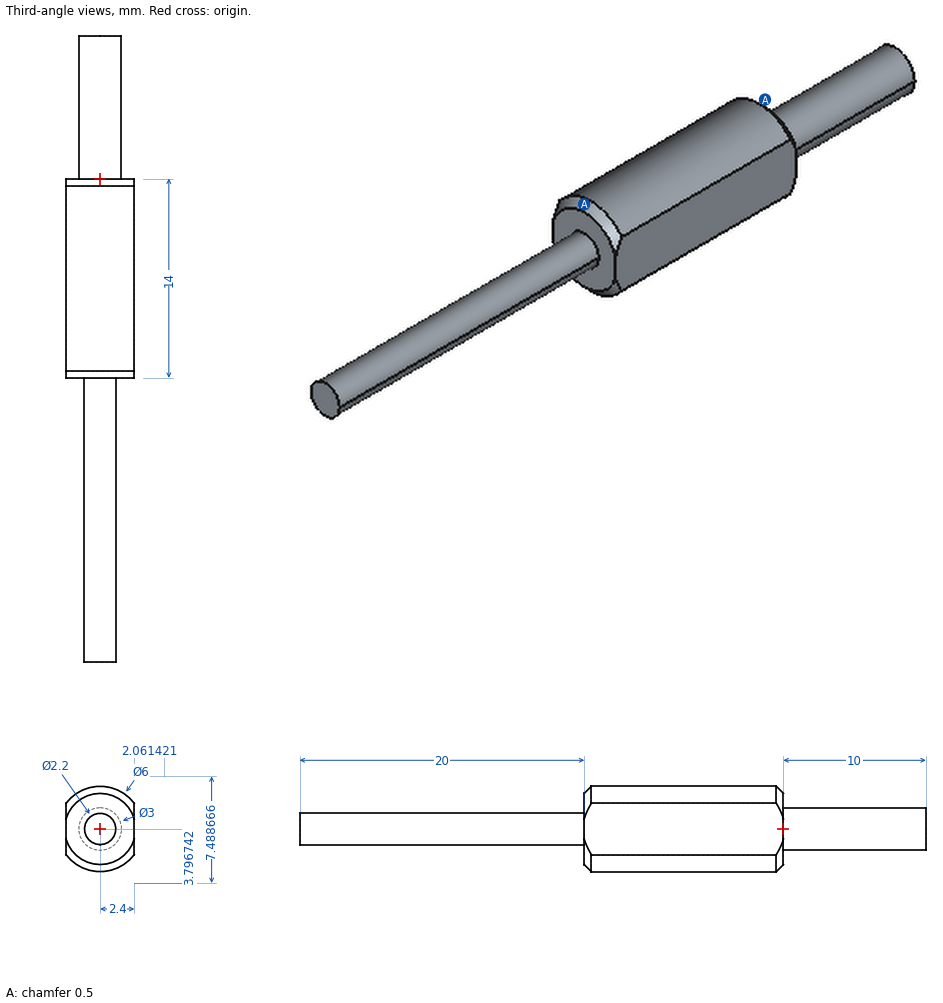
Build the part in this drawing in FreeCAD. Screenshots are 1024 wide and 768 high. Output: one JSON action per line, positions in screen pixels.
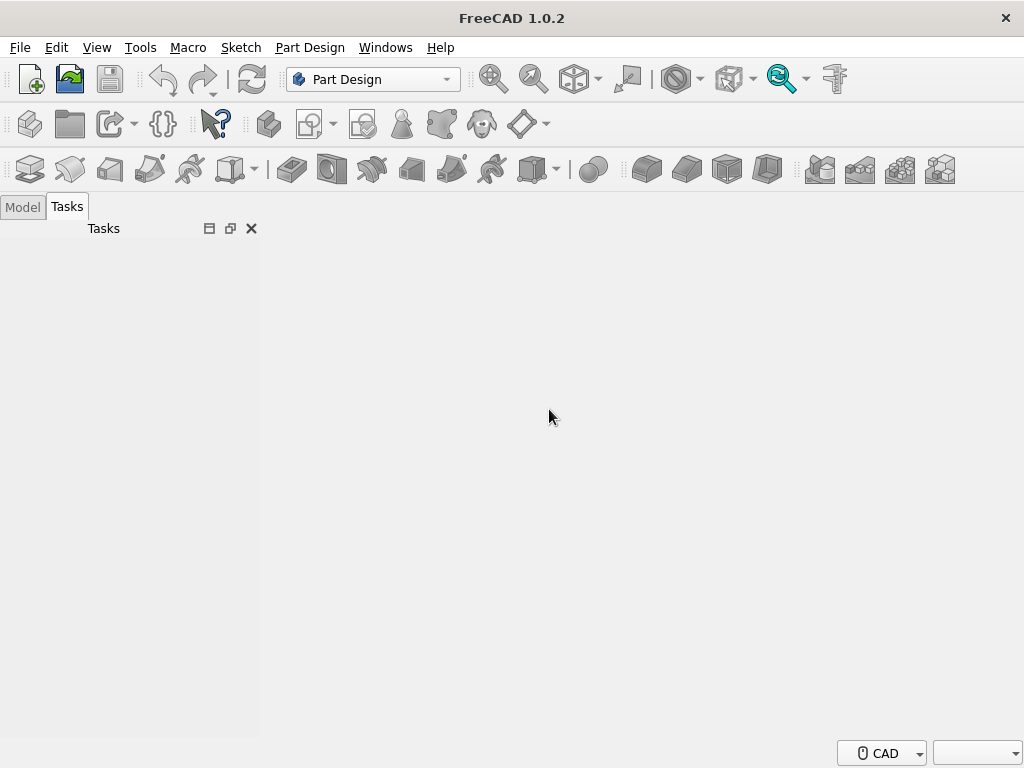
{"action": "key", "text": "ctrl+n"}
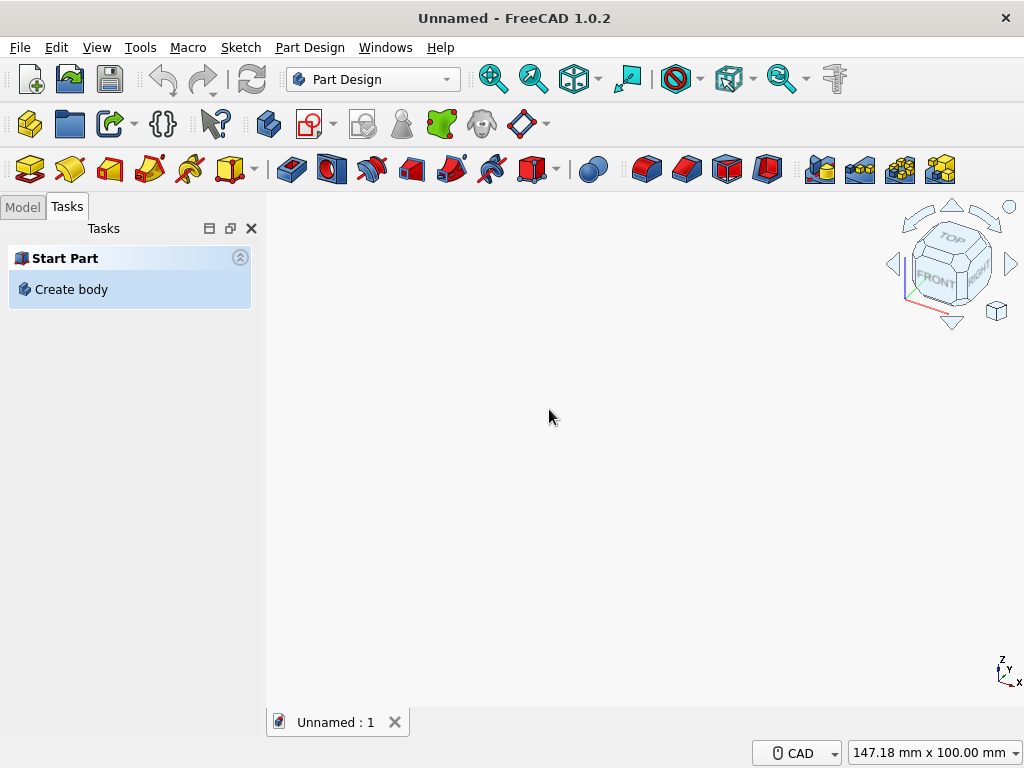
{"action": "left_click", "coordinate": [310, 124]}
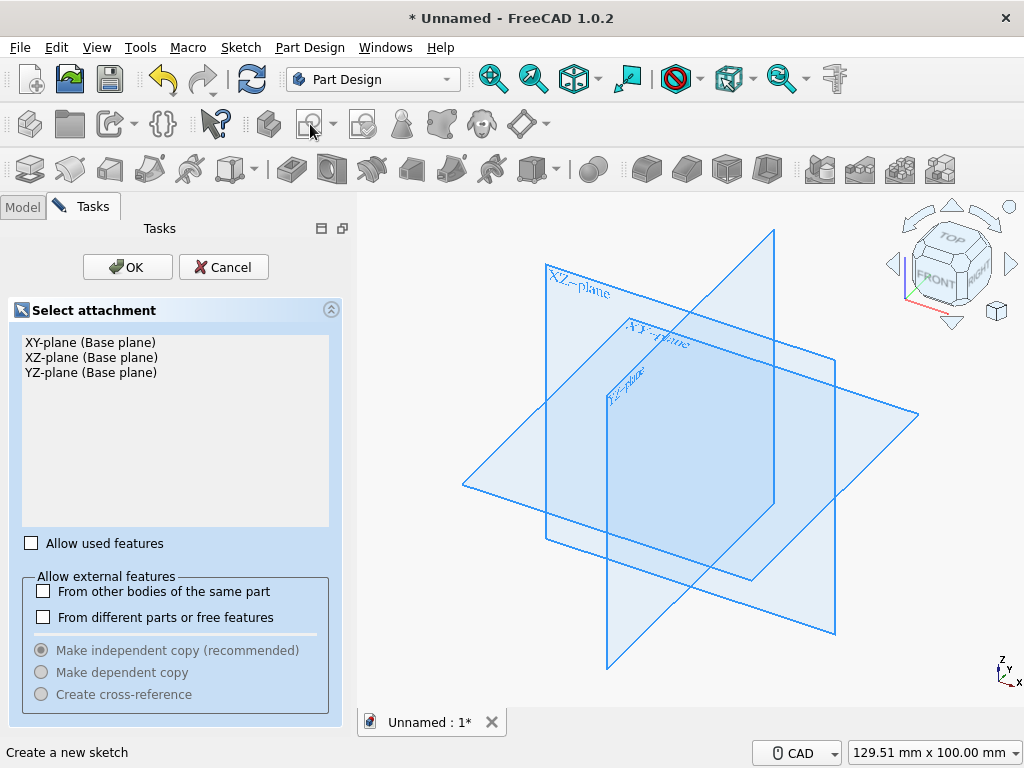
{"action": "left_click", "coordinate": [82, 358]}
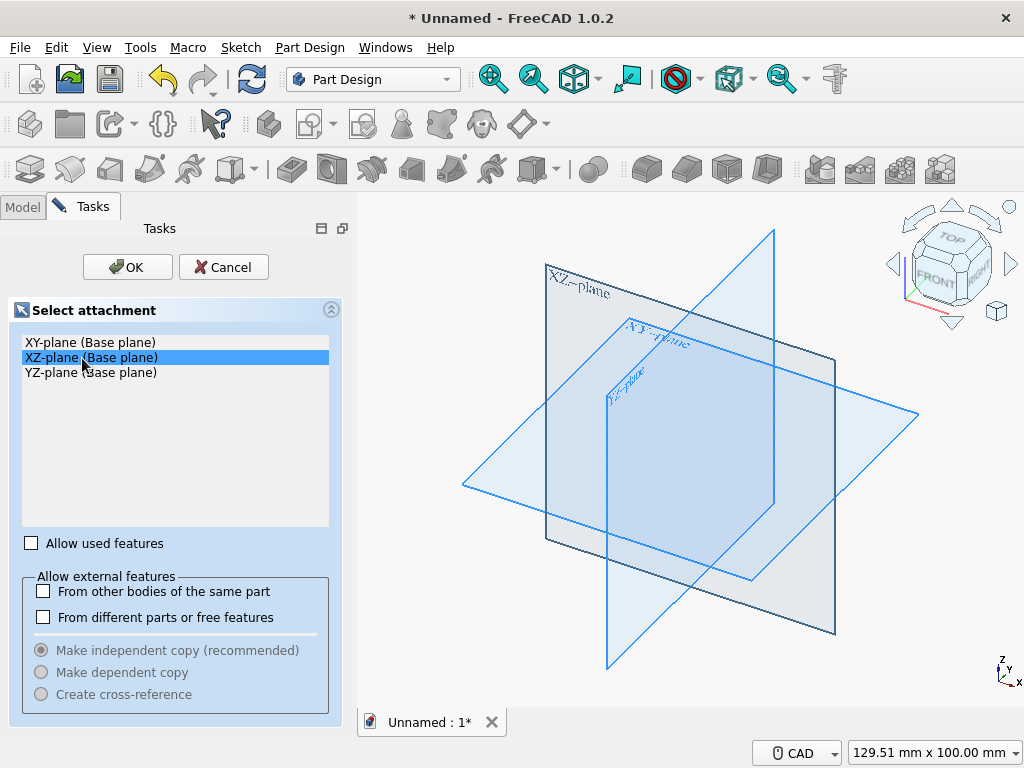
{"action": "left_click", "coordinate": [128, 267]}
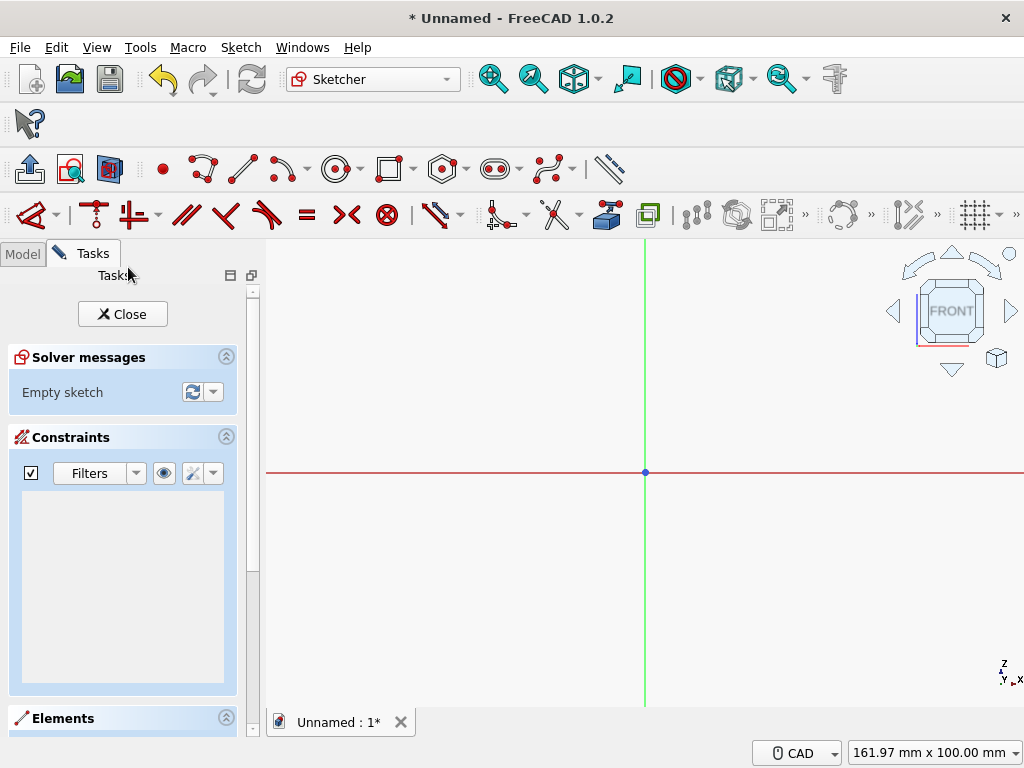
{"action": "scroll", "coordinate": [649, 473], "scroll_direction": "up", "scroll_amount": 15}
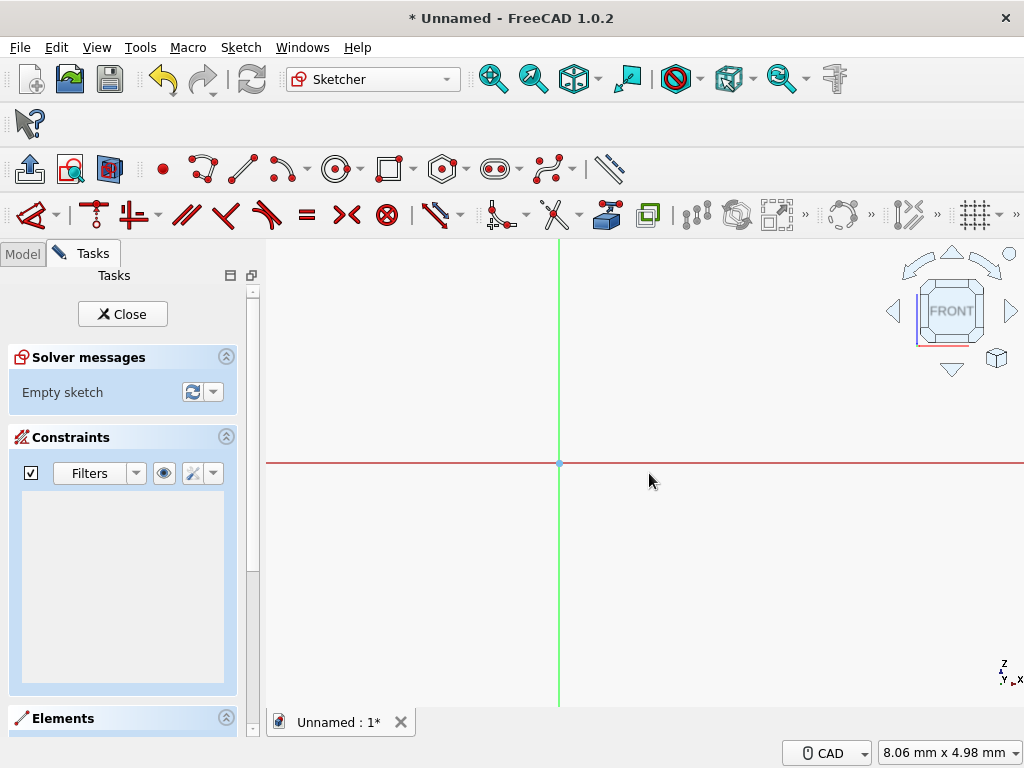
{"action": "left_click", "coordinate": [336, 170]}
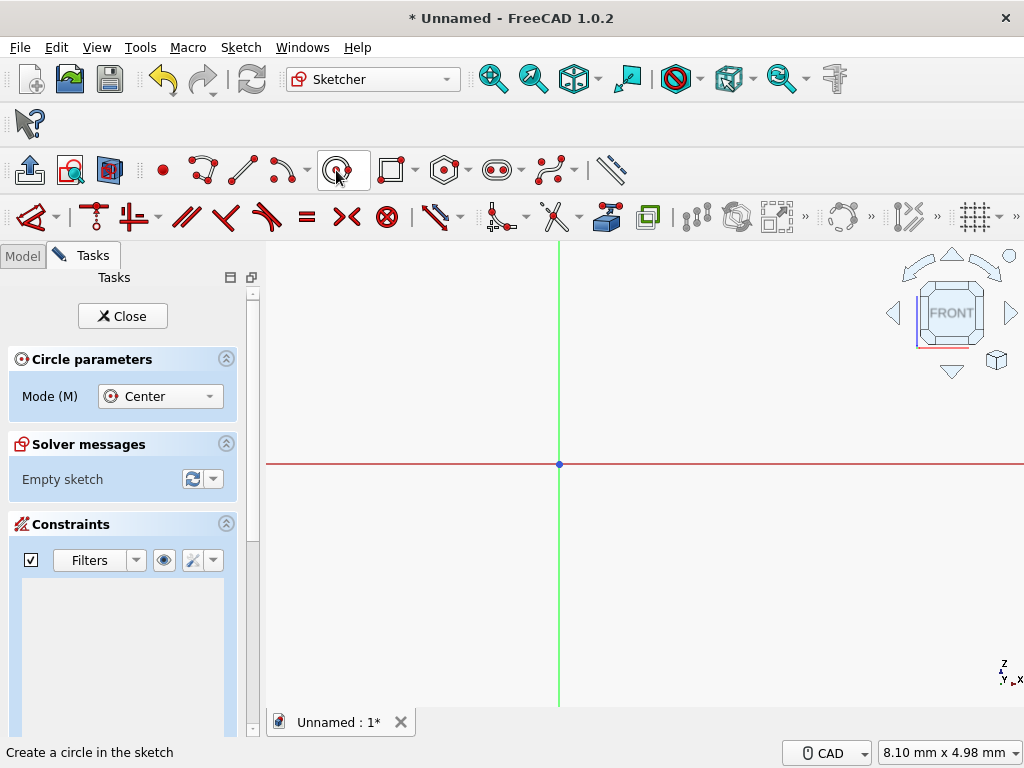
{"action": "left_click", "coordinate": [559, 464]}
{"action": "left_click", "coordinate": [659, 365]}
{"action": "key", "text": "Escape"}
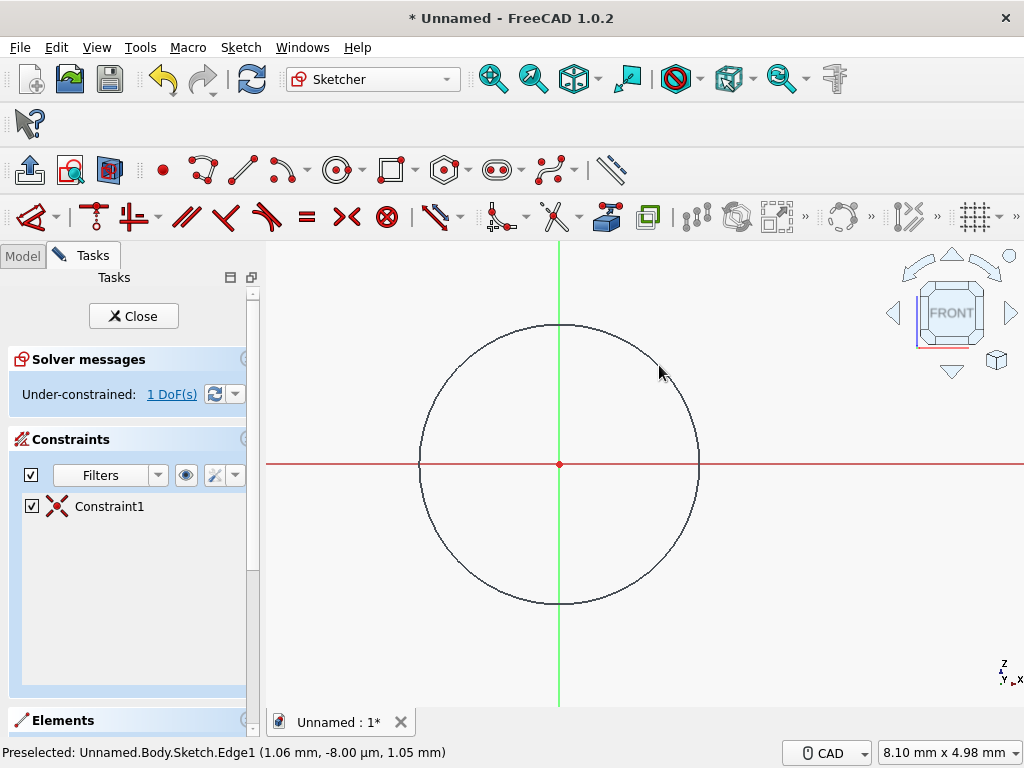
{"action": "left_click", "coordinate": [32, 218]}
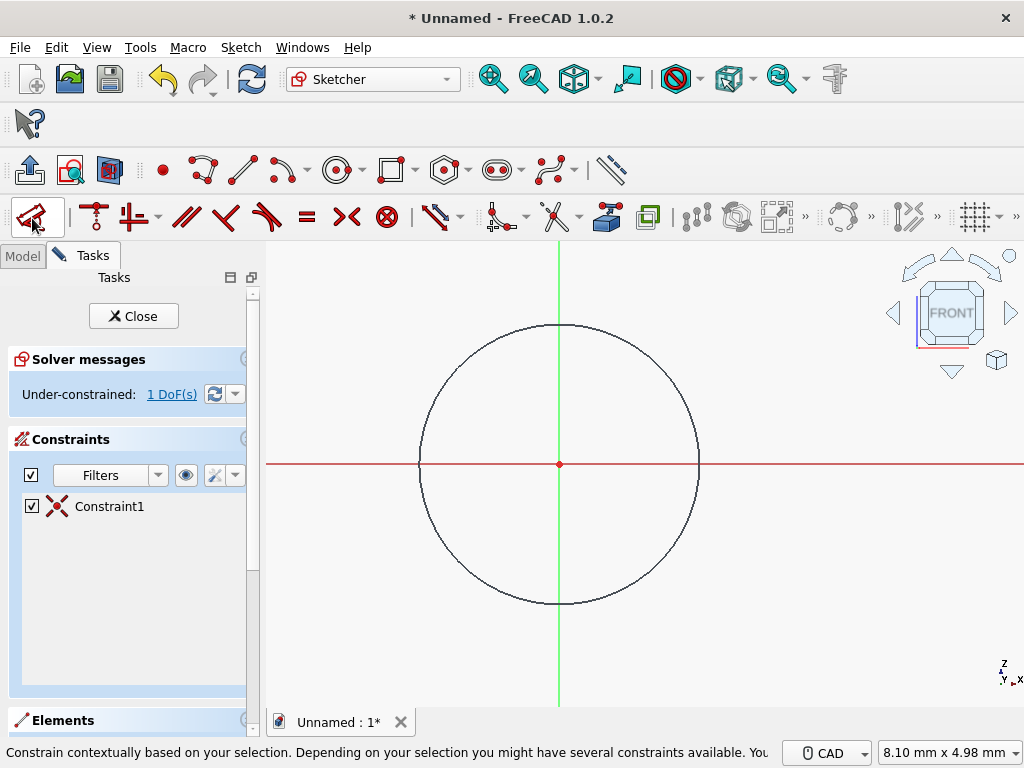
{"action": "left_click", "coordinate": [658, 365]}
{"action": "left_click", "coordinate": [681, 342]}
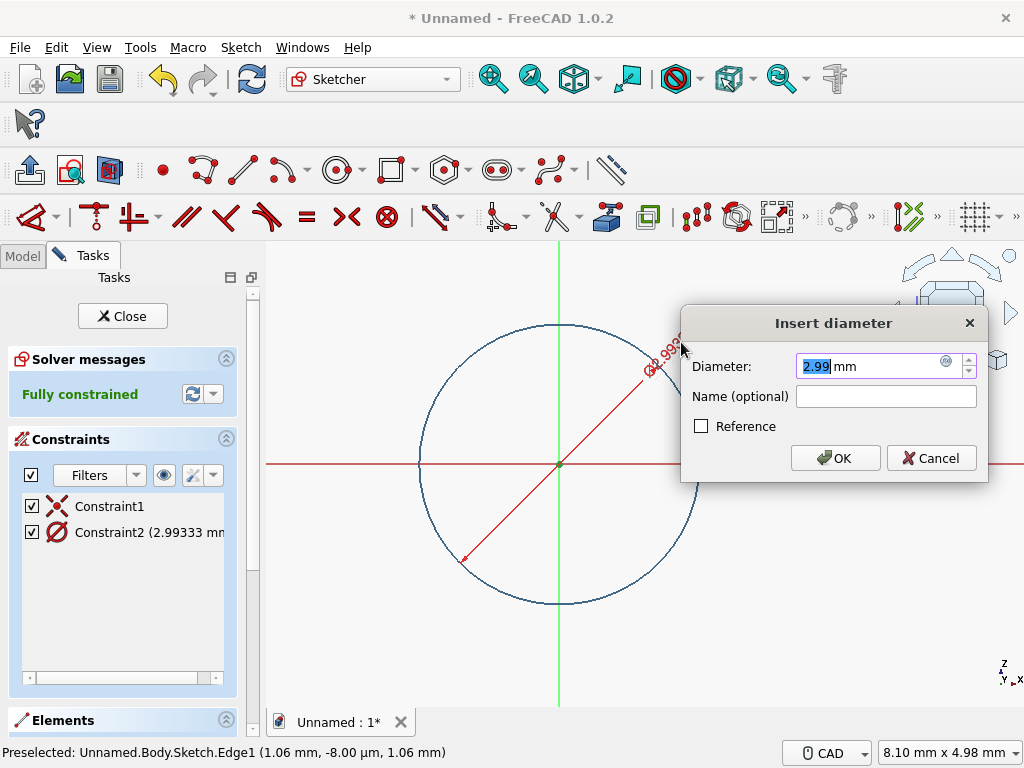
{"action": "type", "text": "3"}
{"action": "key", "text": "Return"}
{"action": "key", "text": "Escape"}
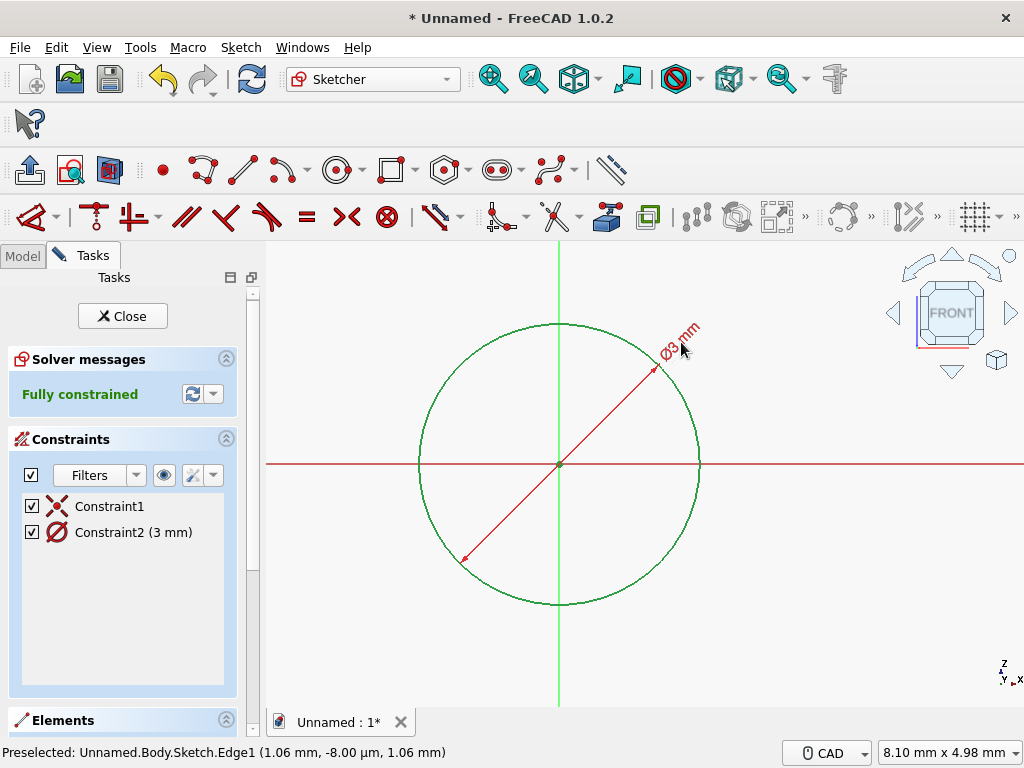
{"action": "left_click", "coordinate": [123, 316]}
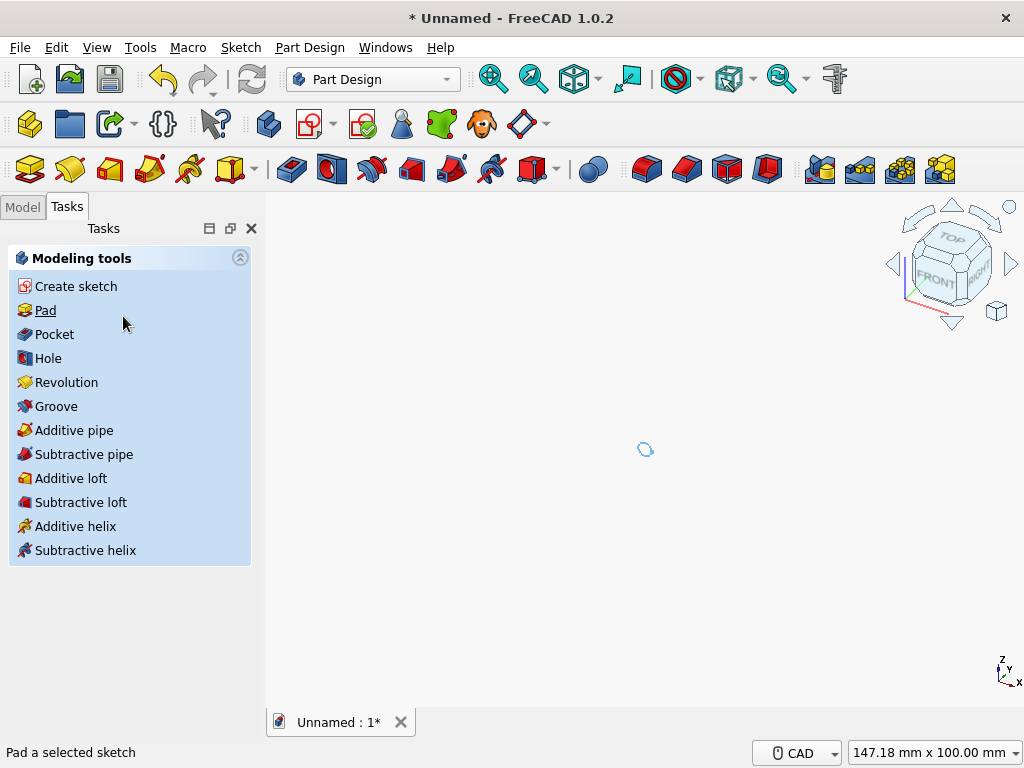
{"action": "left_click", "coordinate": [30, 170]}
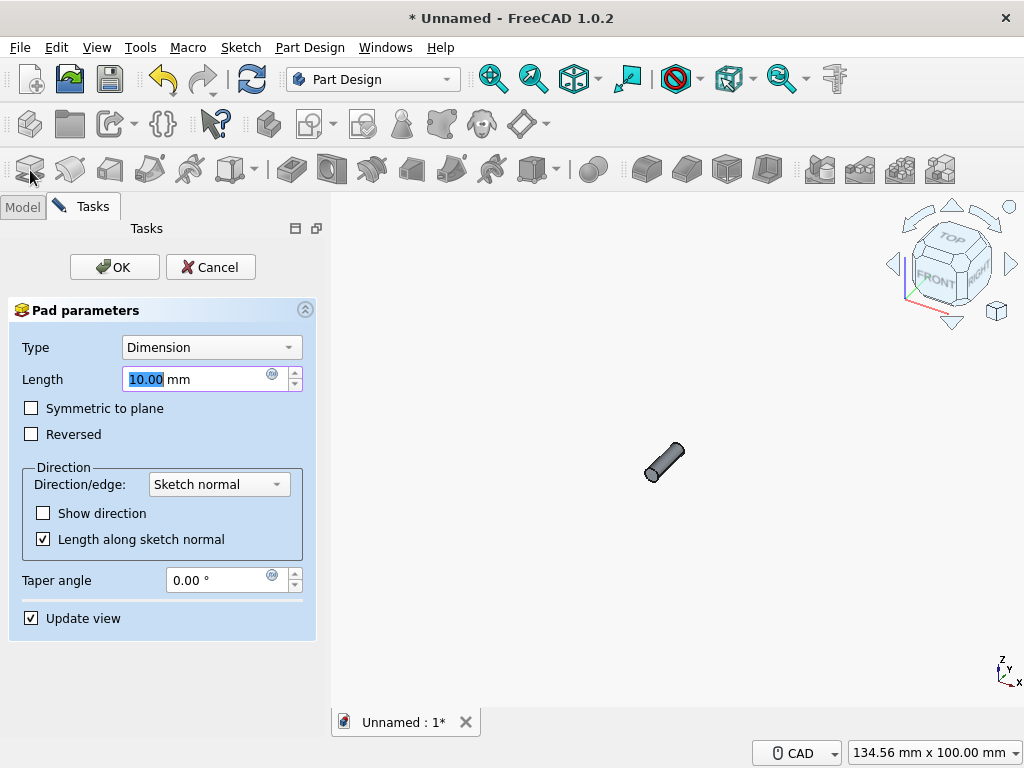
{"action": "type", "text": "10"}
{"action": "key", "text": "Tab"}